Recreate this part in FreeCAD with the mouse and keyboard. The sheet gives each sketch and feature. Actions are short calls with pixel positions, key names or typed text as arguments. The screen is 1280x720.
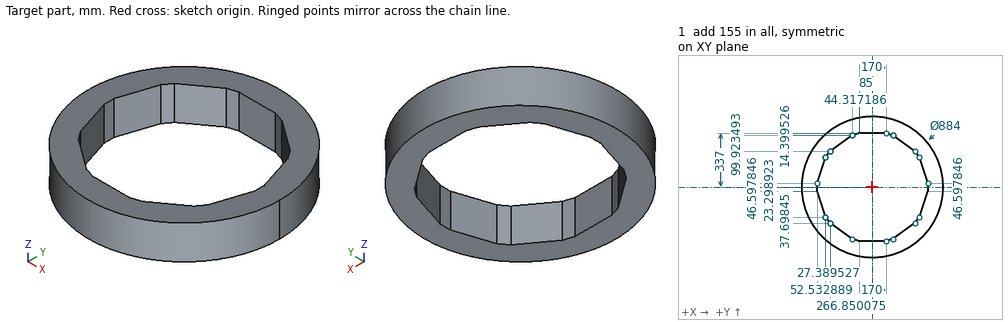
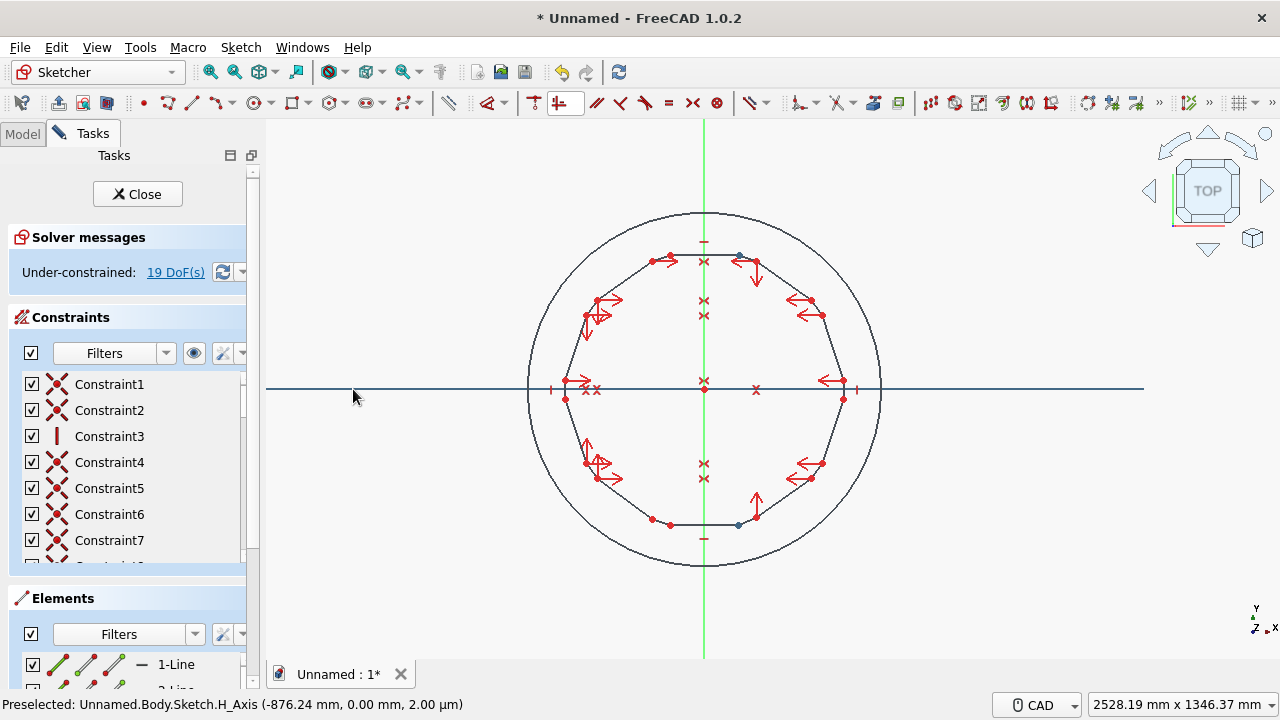
key(s)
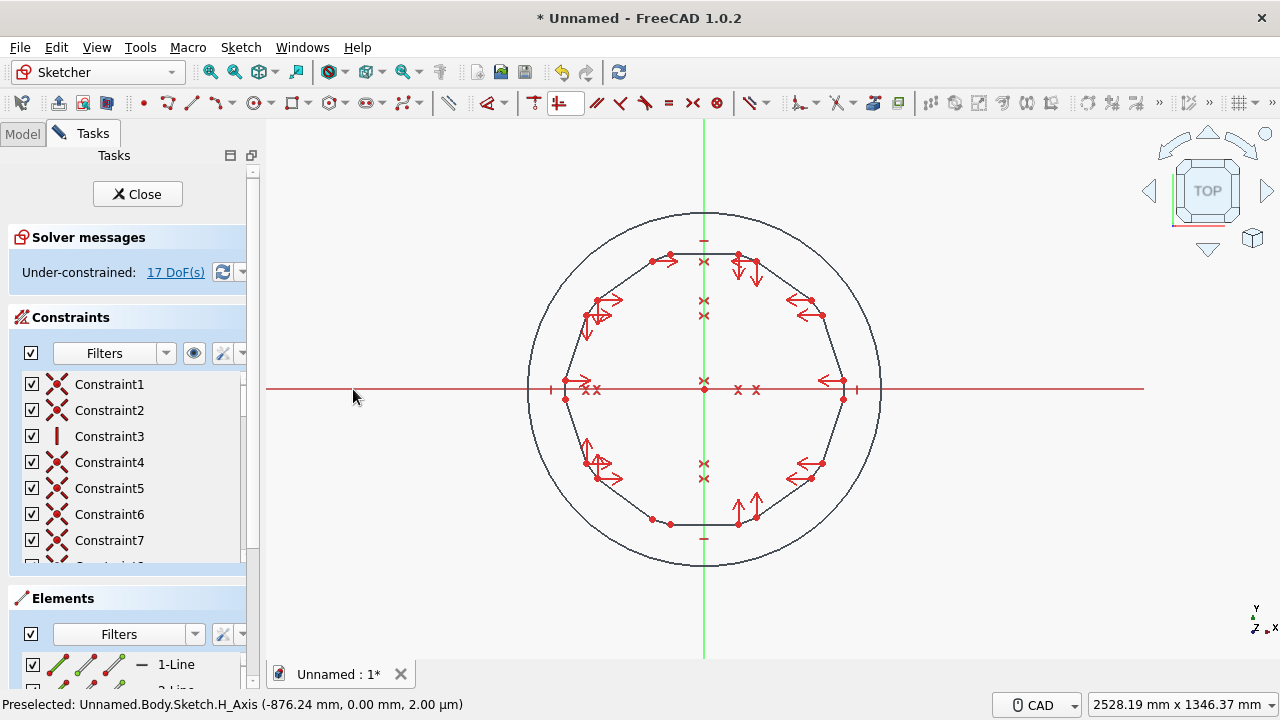
click(652, 261)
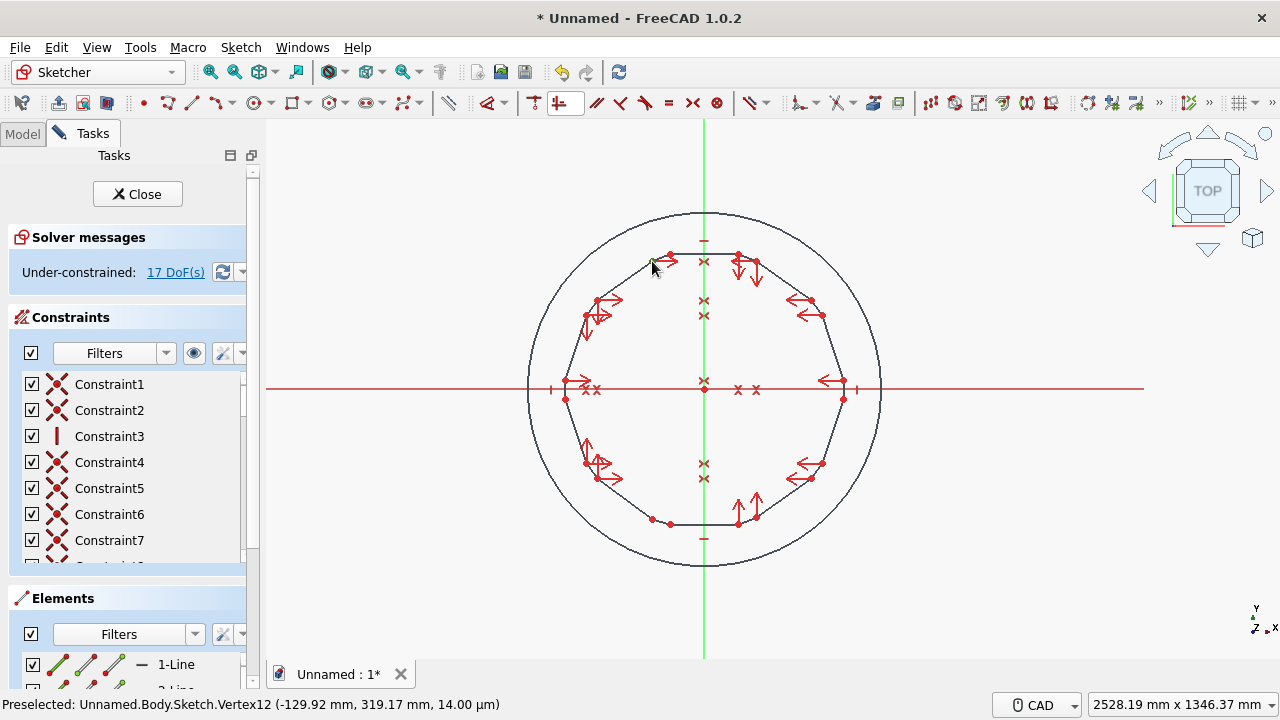
click(653, 519)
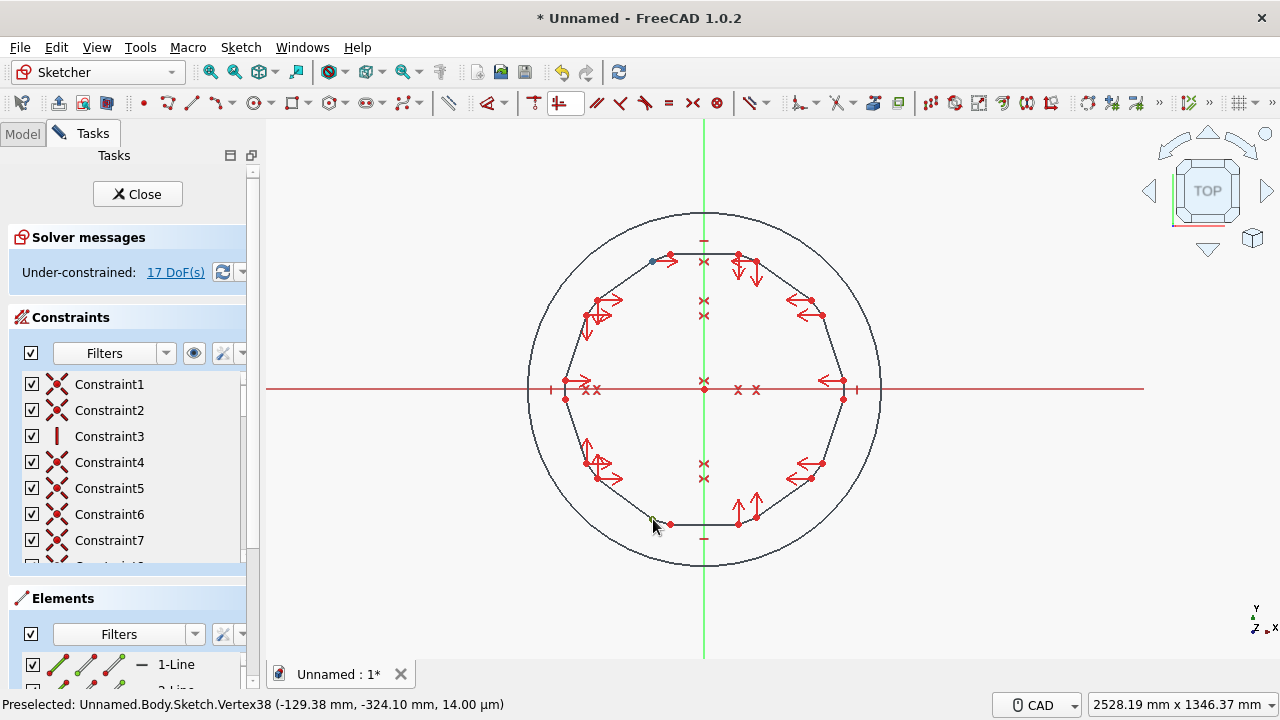
click(353, 389)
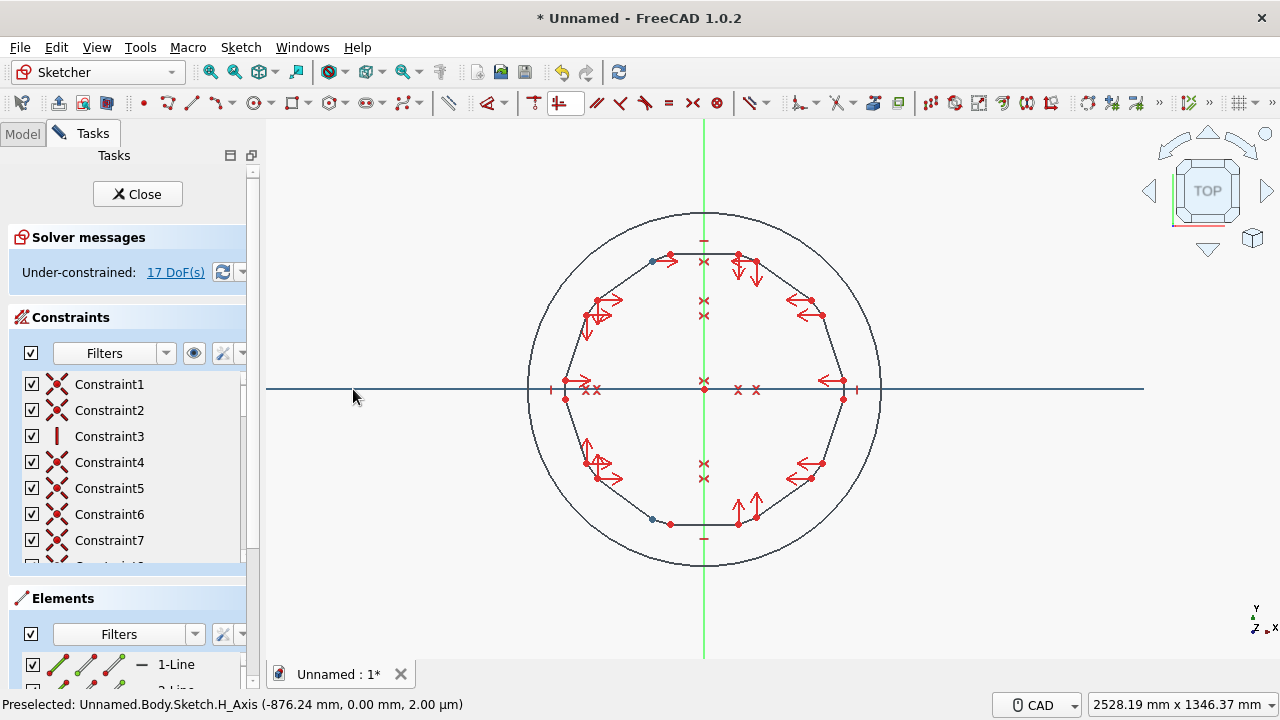
key(s)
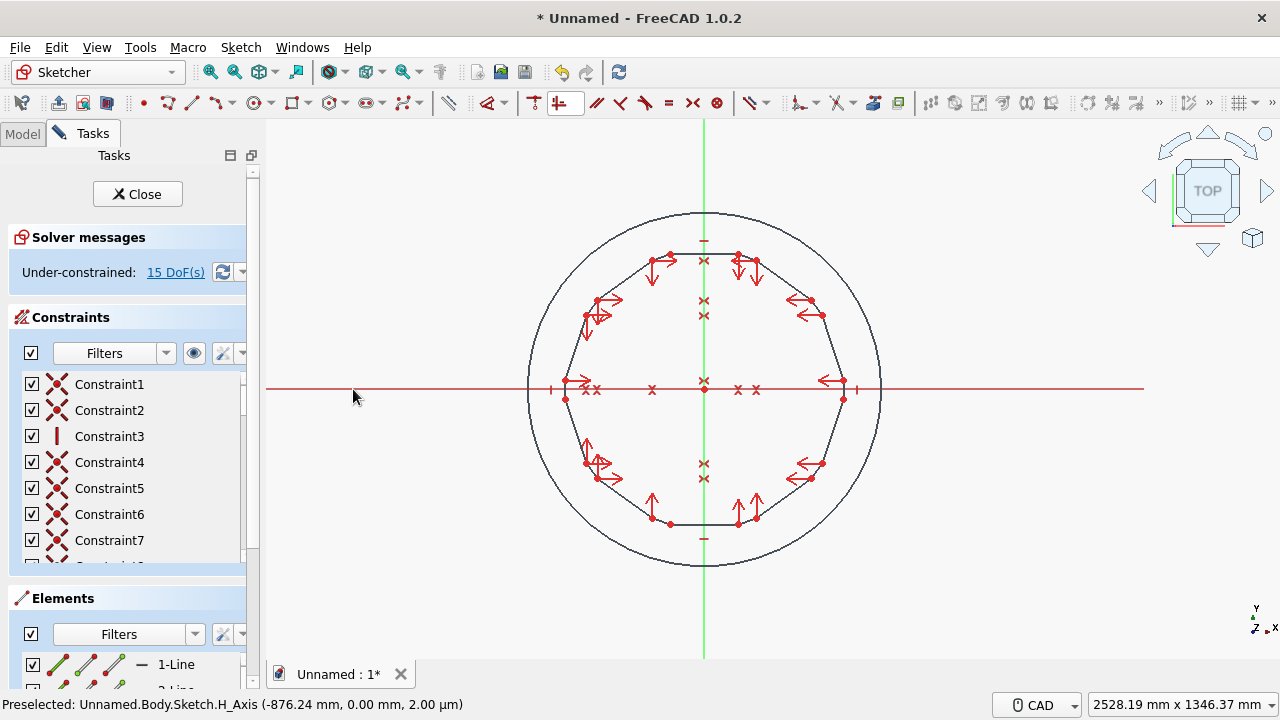
key(d)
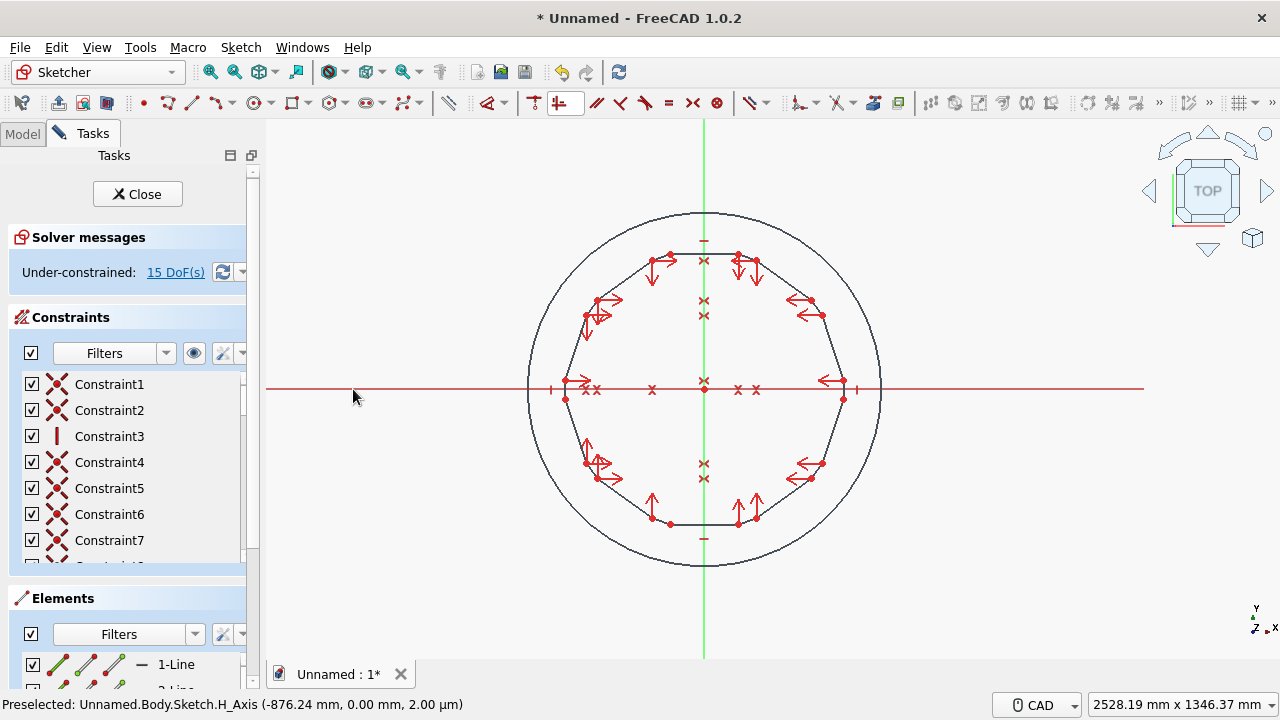
click(829, 264)
click(852, 241)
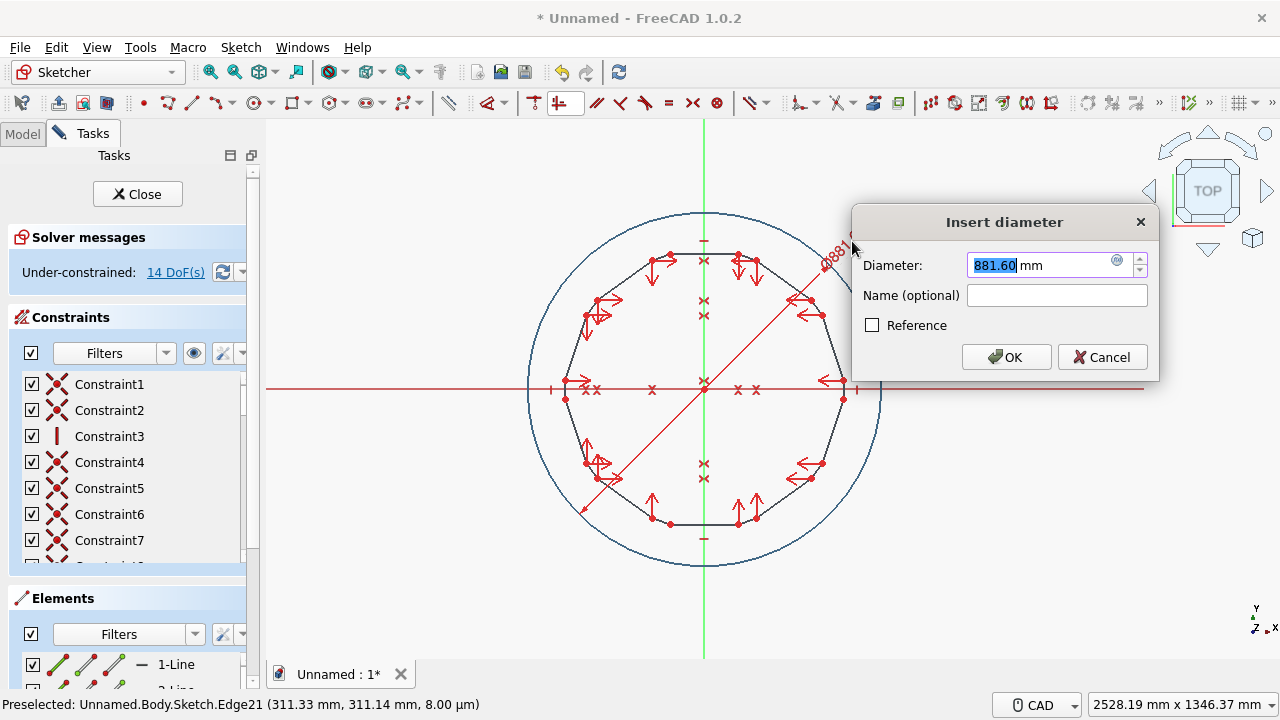
text(884)
key(Return)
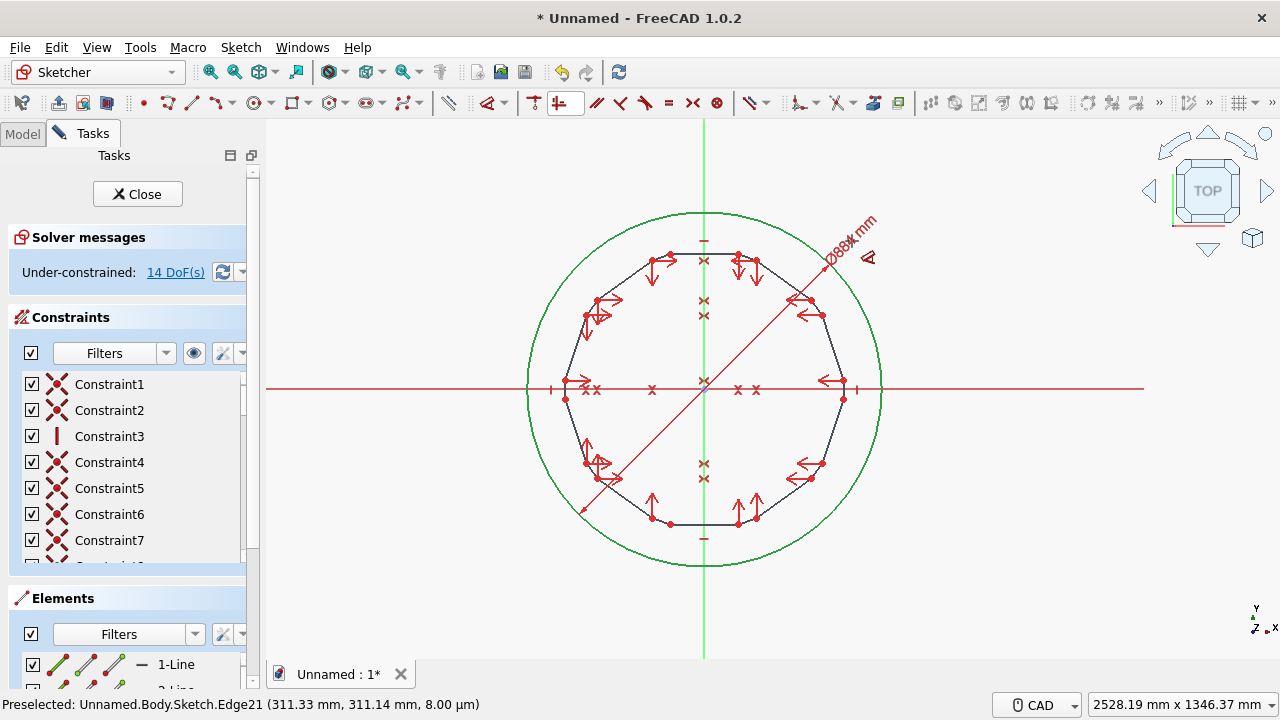
click(691, 254)
click(689, 288)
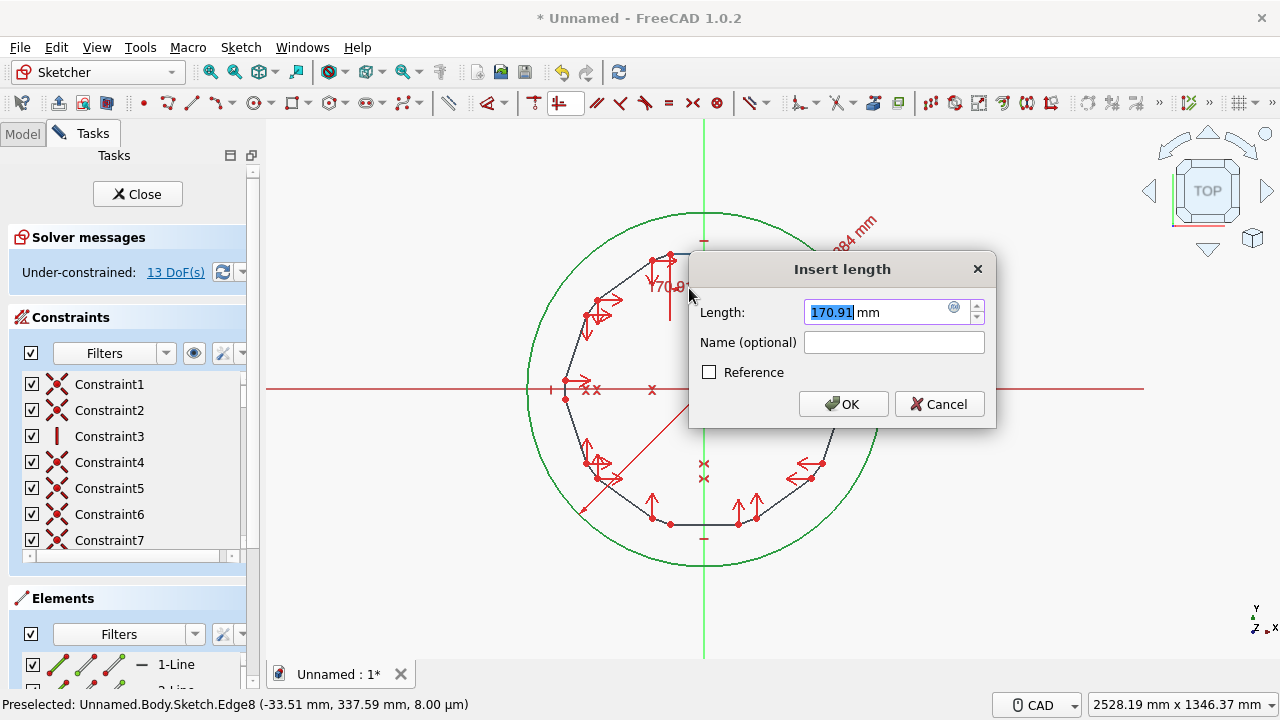
text(170)
key(Return)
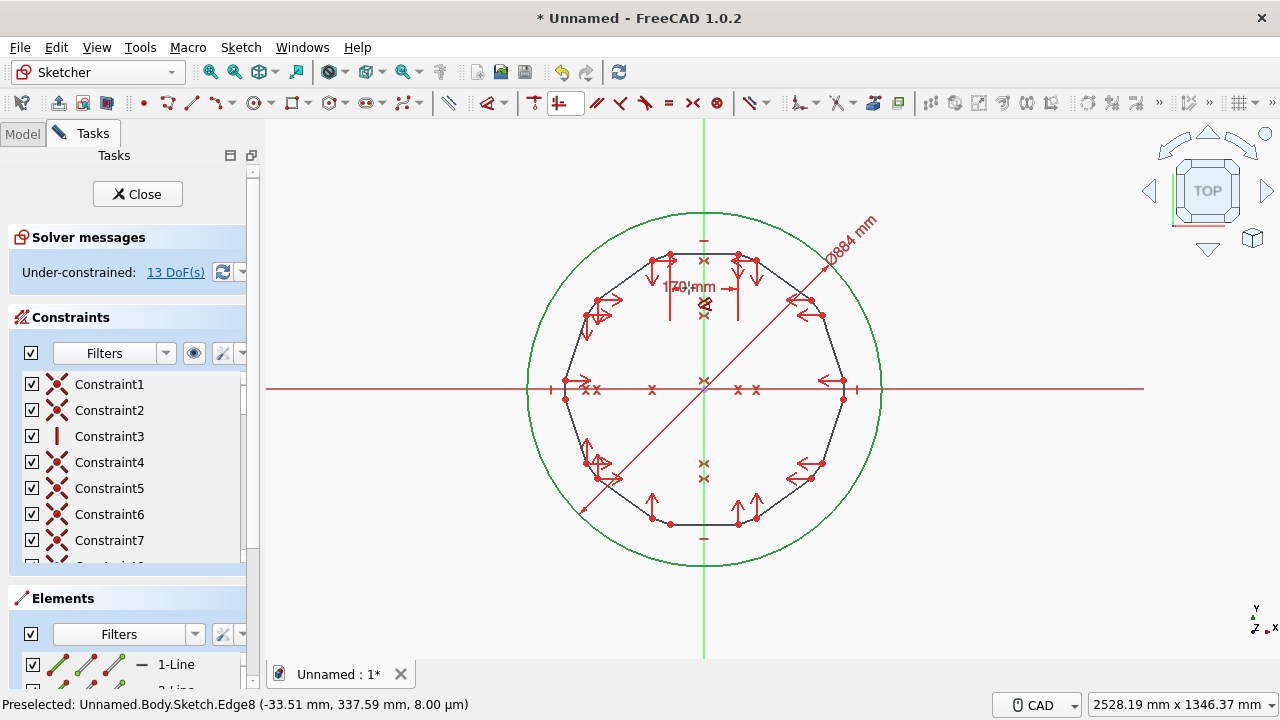
click(718, 525)
click(689, 491)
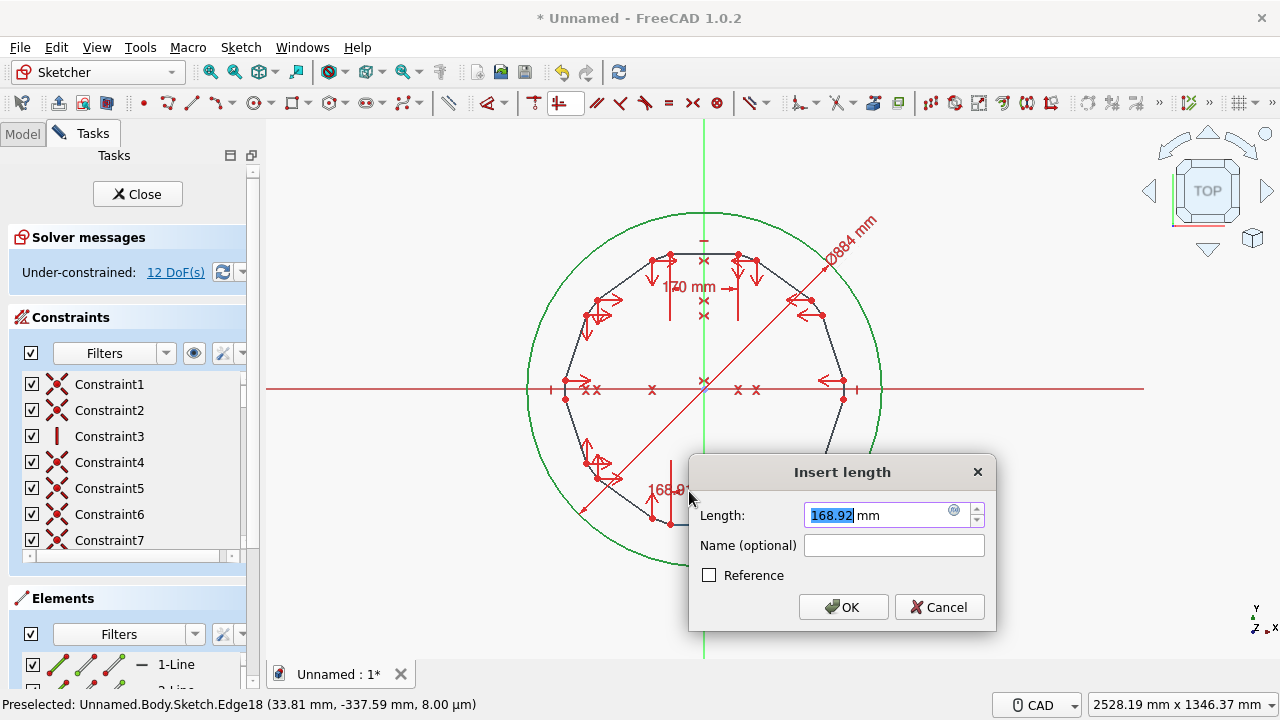
text(170)
key(Return)